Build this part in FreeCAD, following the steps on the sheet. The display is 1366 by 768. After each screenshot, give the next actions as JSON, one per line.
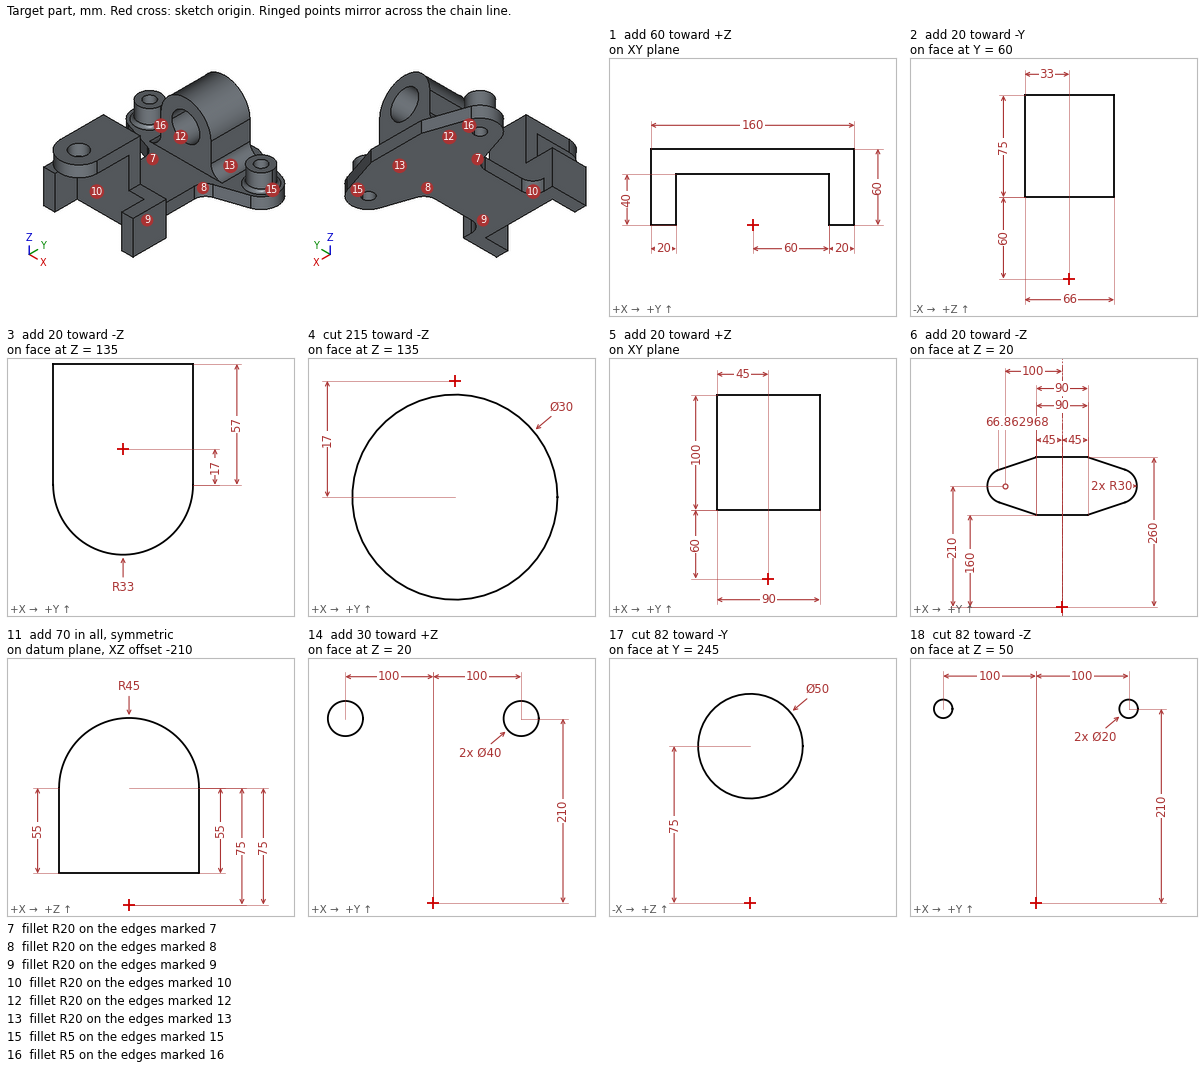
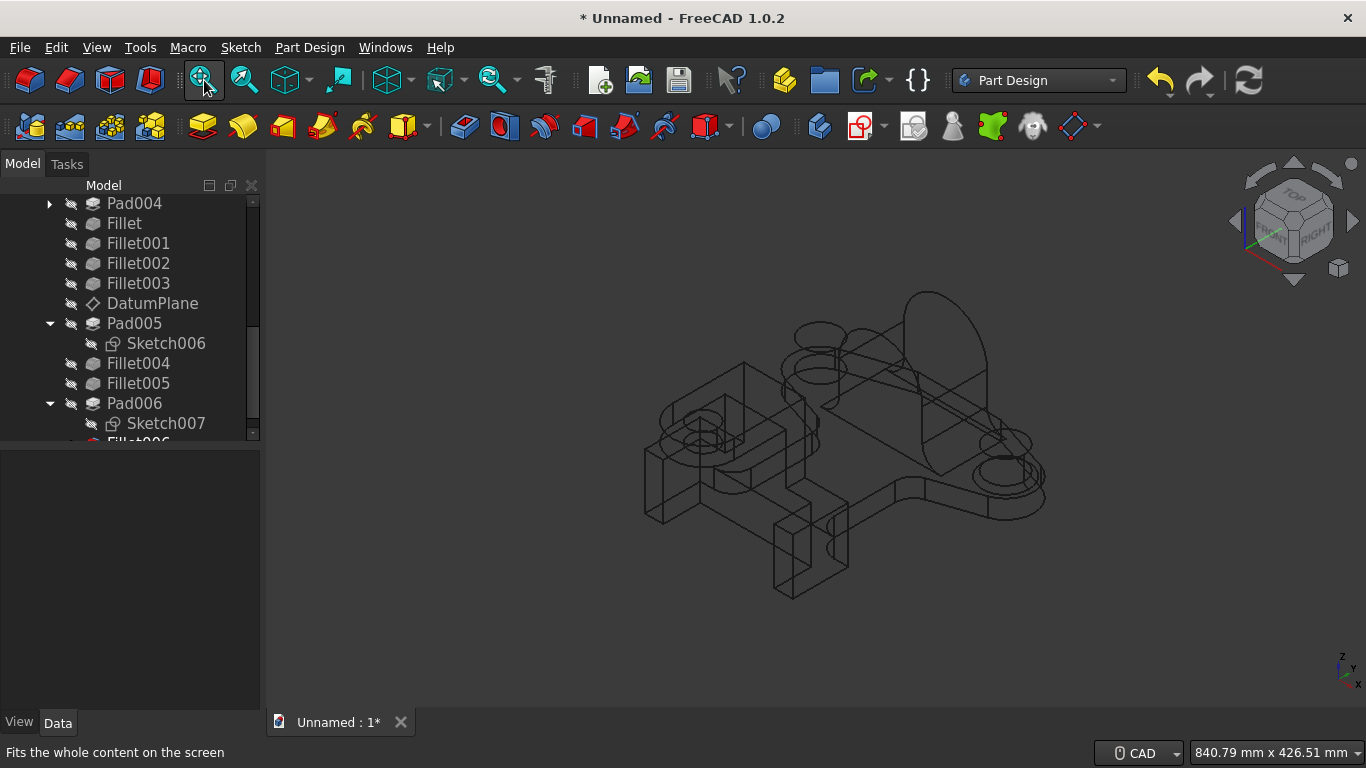
{"action": "left_click", "coordinate": [802, 358]}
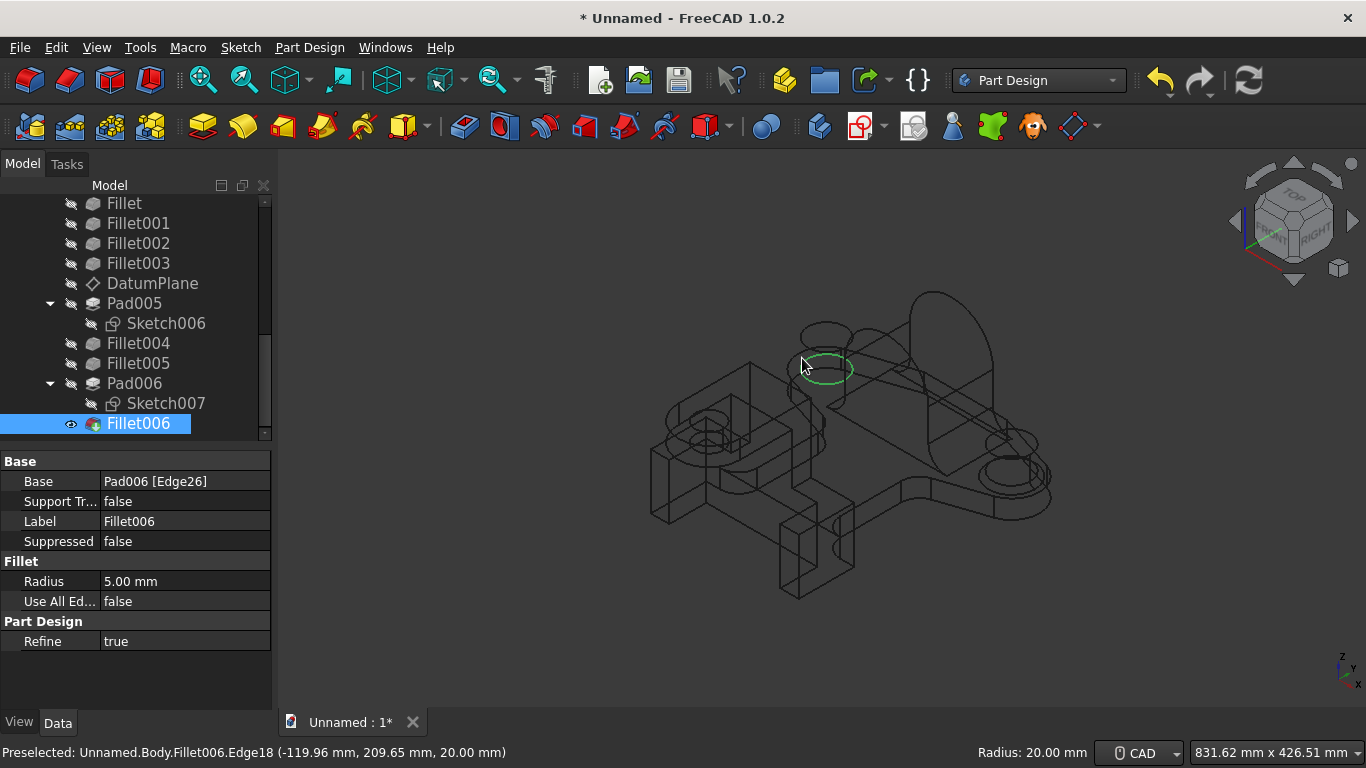
{"action": "key", "text": "v 1"}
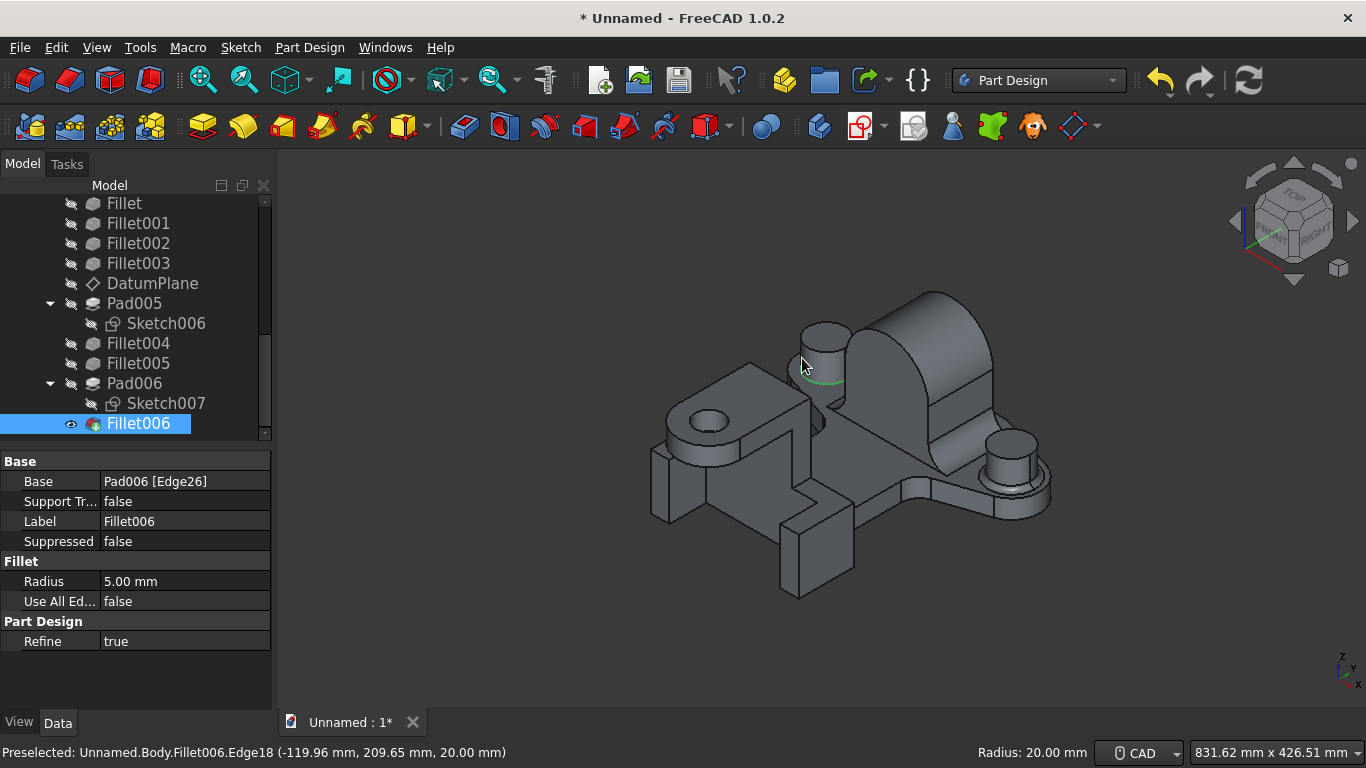
{"action": "left_click", "coordinate": [30, 80]}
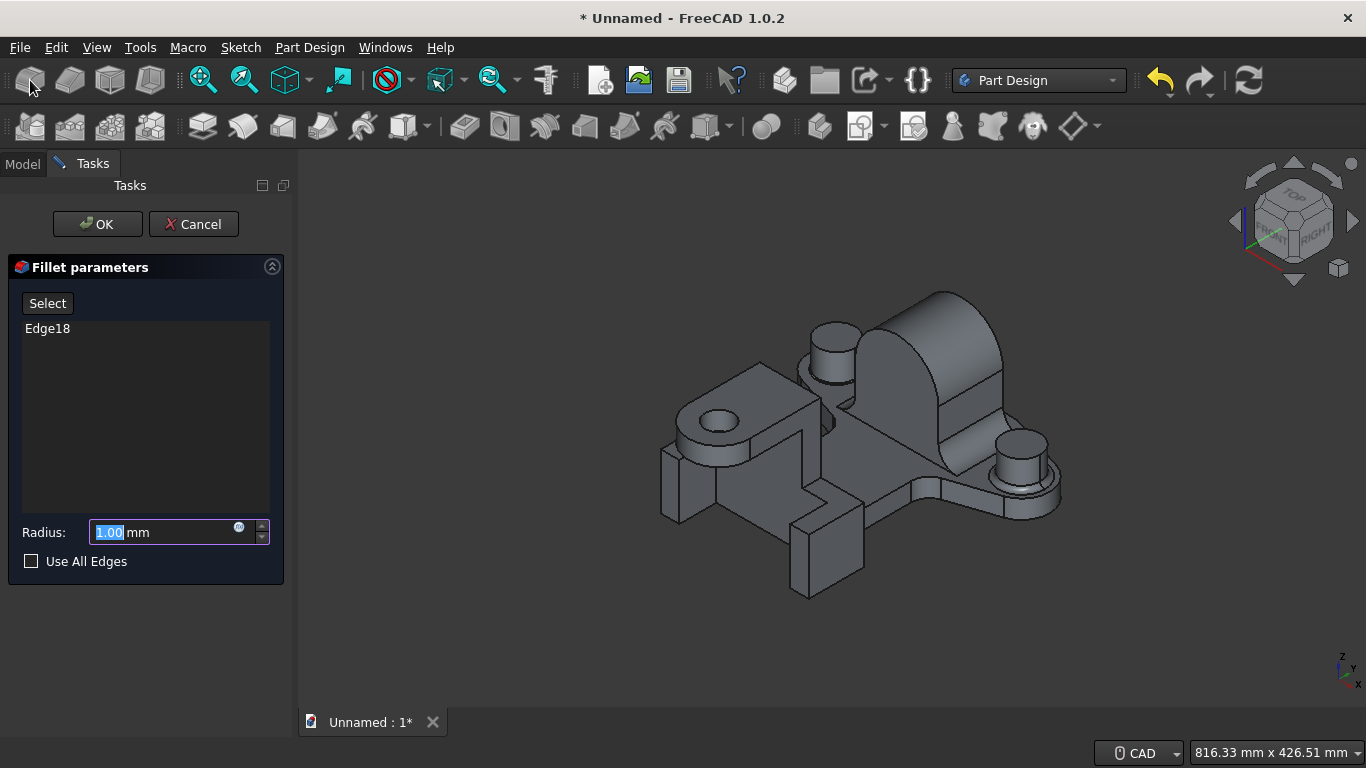
{"action": "type", "text": "5"}
{"action": "key", "text": "Tab"}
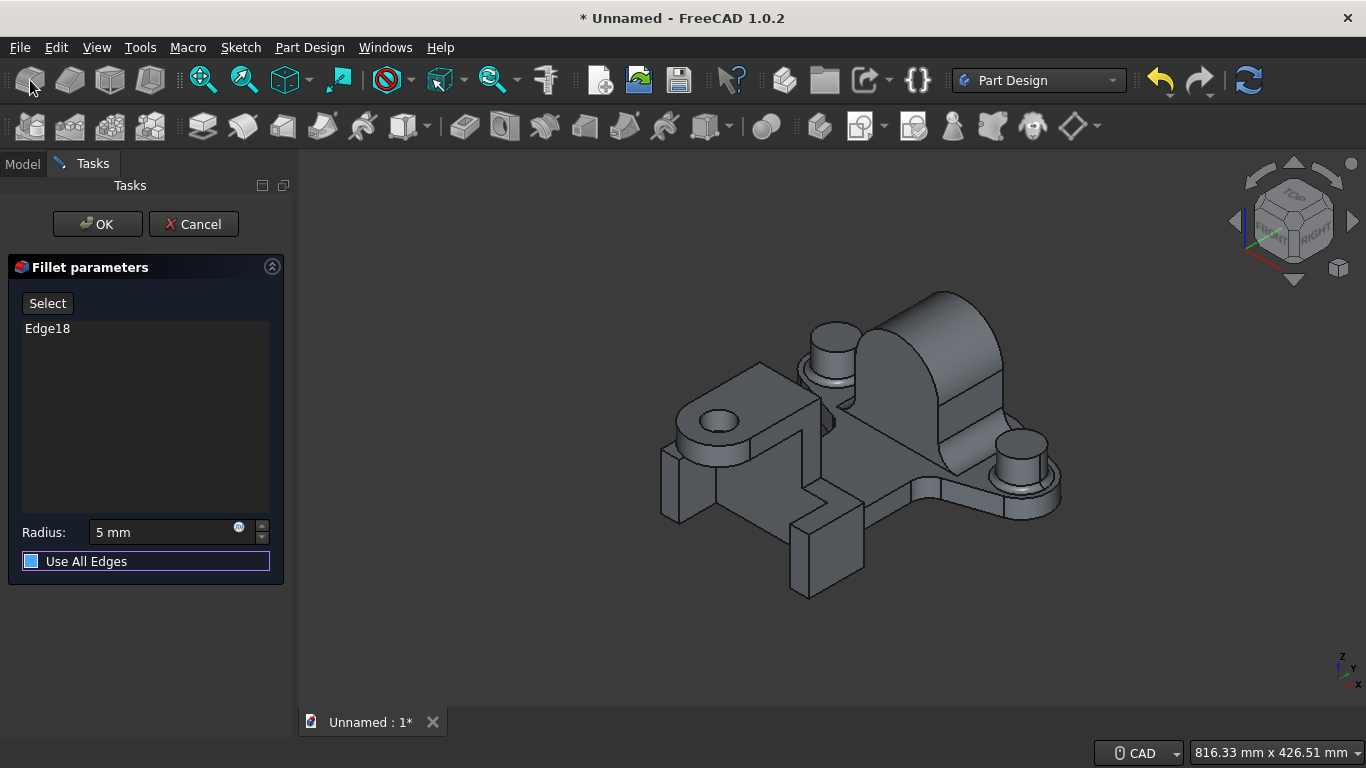
{"action": "left_click", "coordinate": [98, 224]}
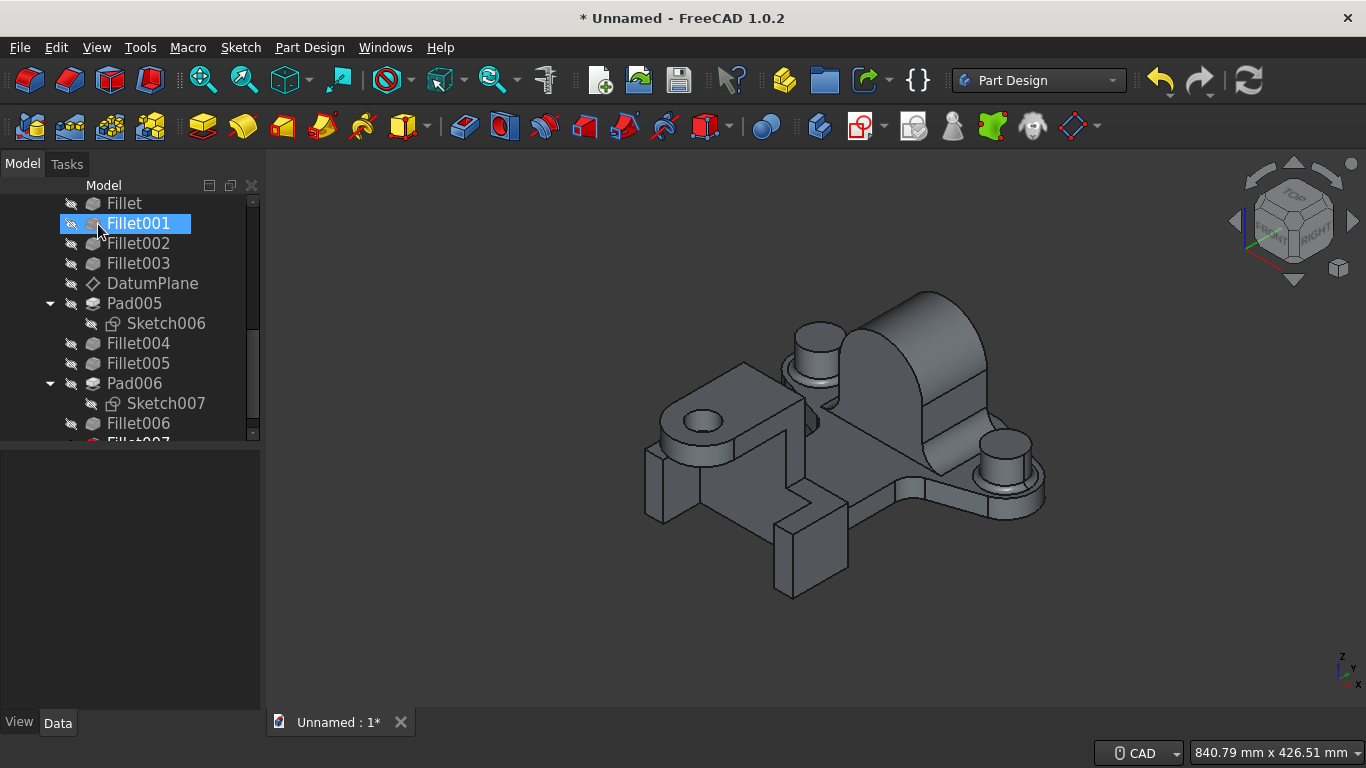
{"action": "key", "text": "4"}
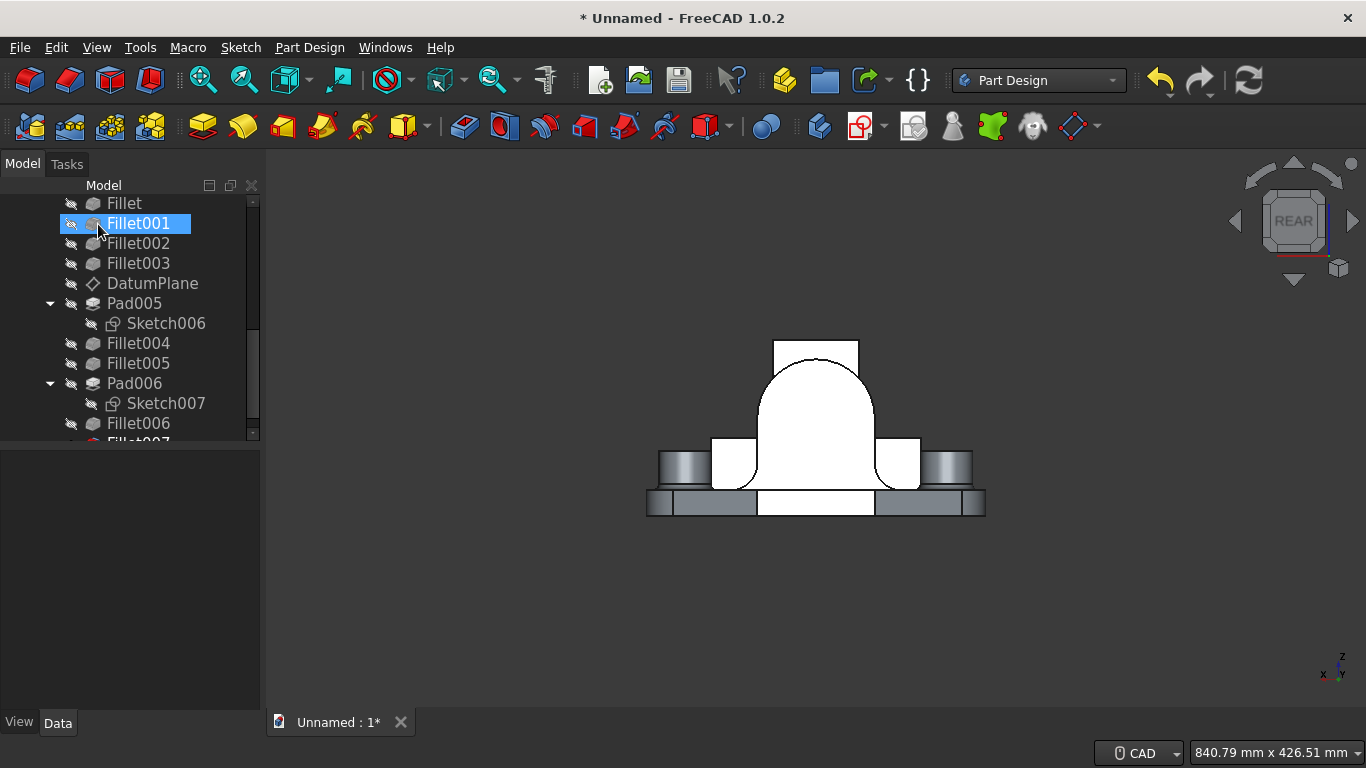
{"action": "key", "text": "v f"}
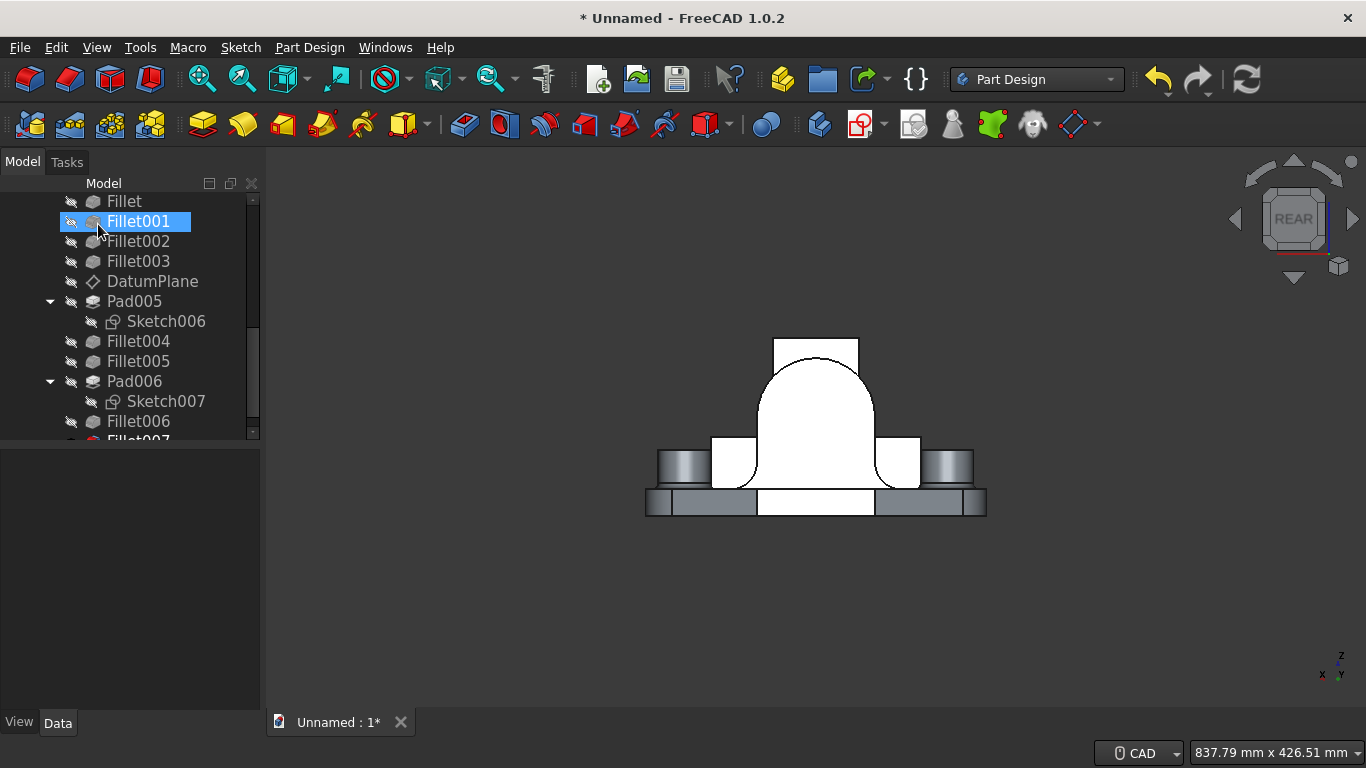
{"action": "left_click", "coordinate": [816, 423]}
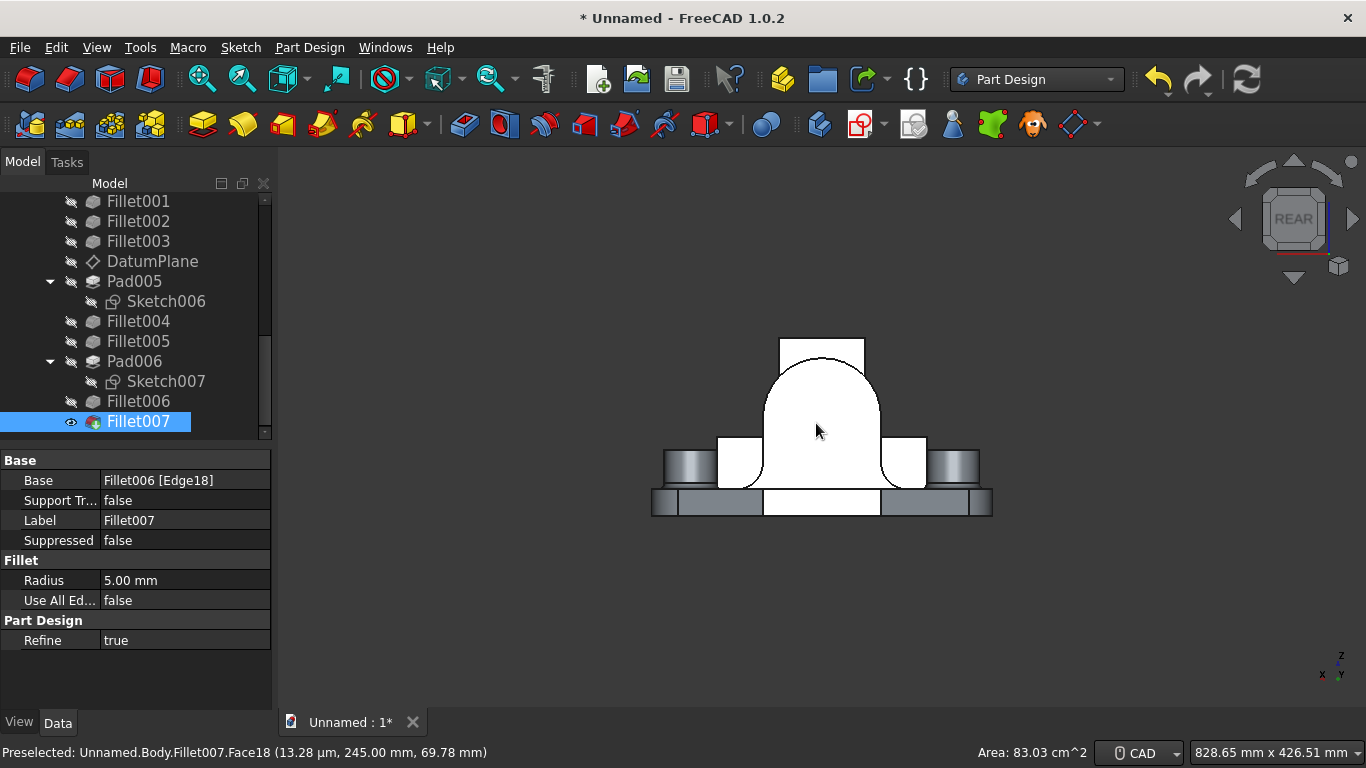
{"action": "left_click", "coordinate": [860, 124]}